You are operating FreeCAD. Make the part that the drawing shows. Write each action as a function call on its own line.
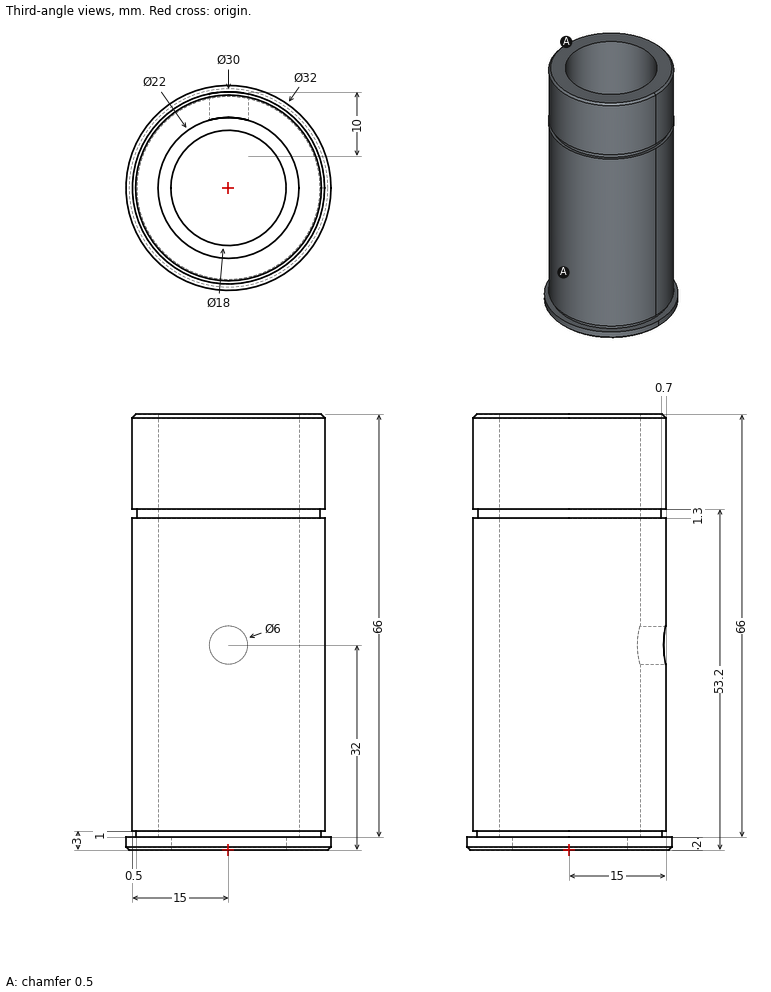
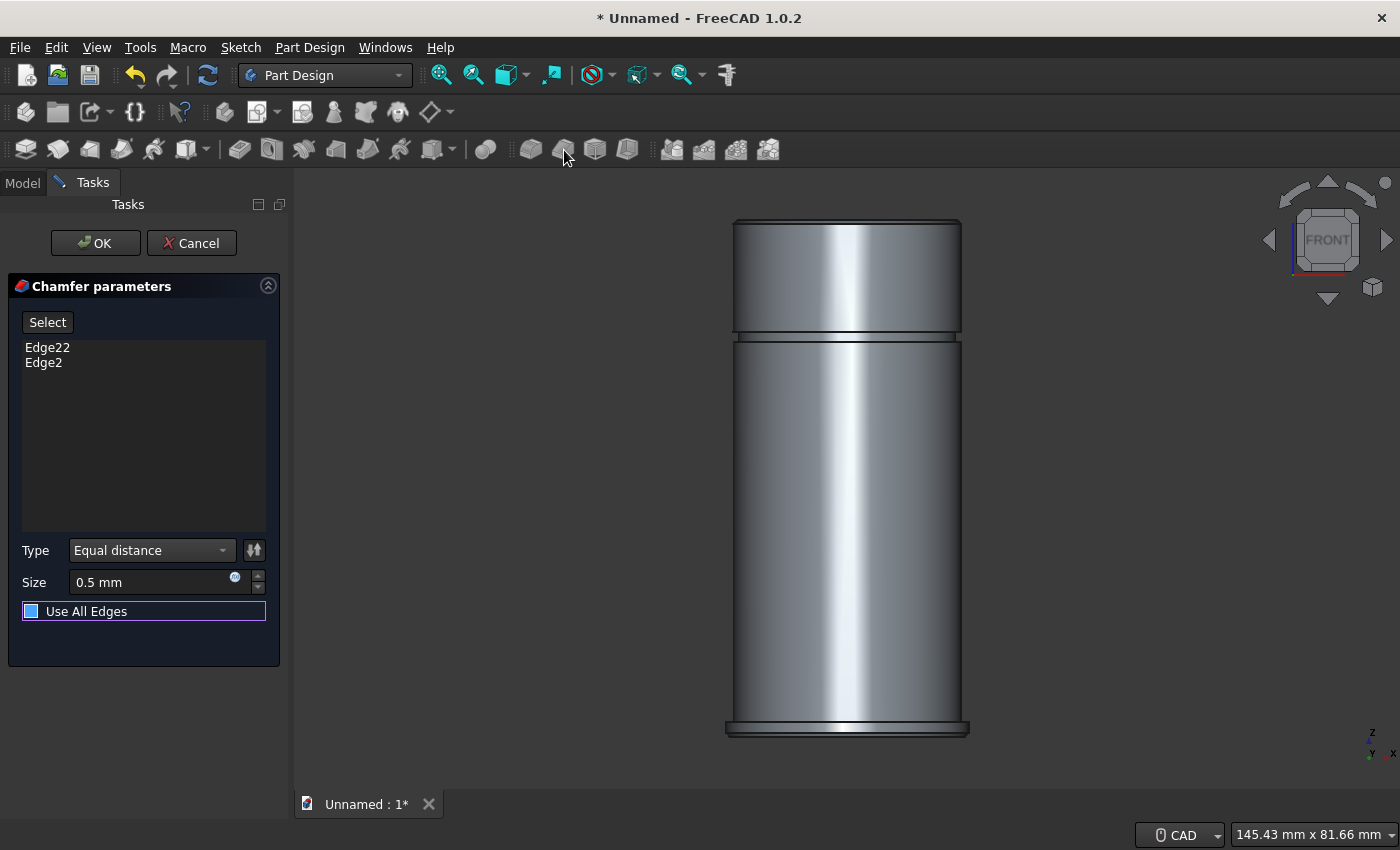
click(96, 243)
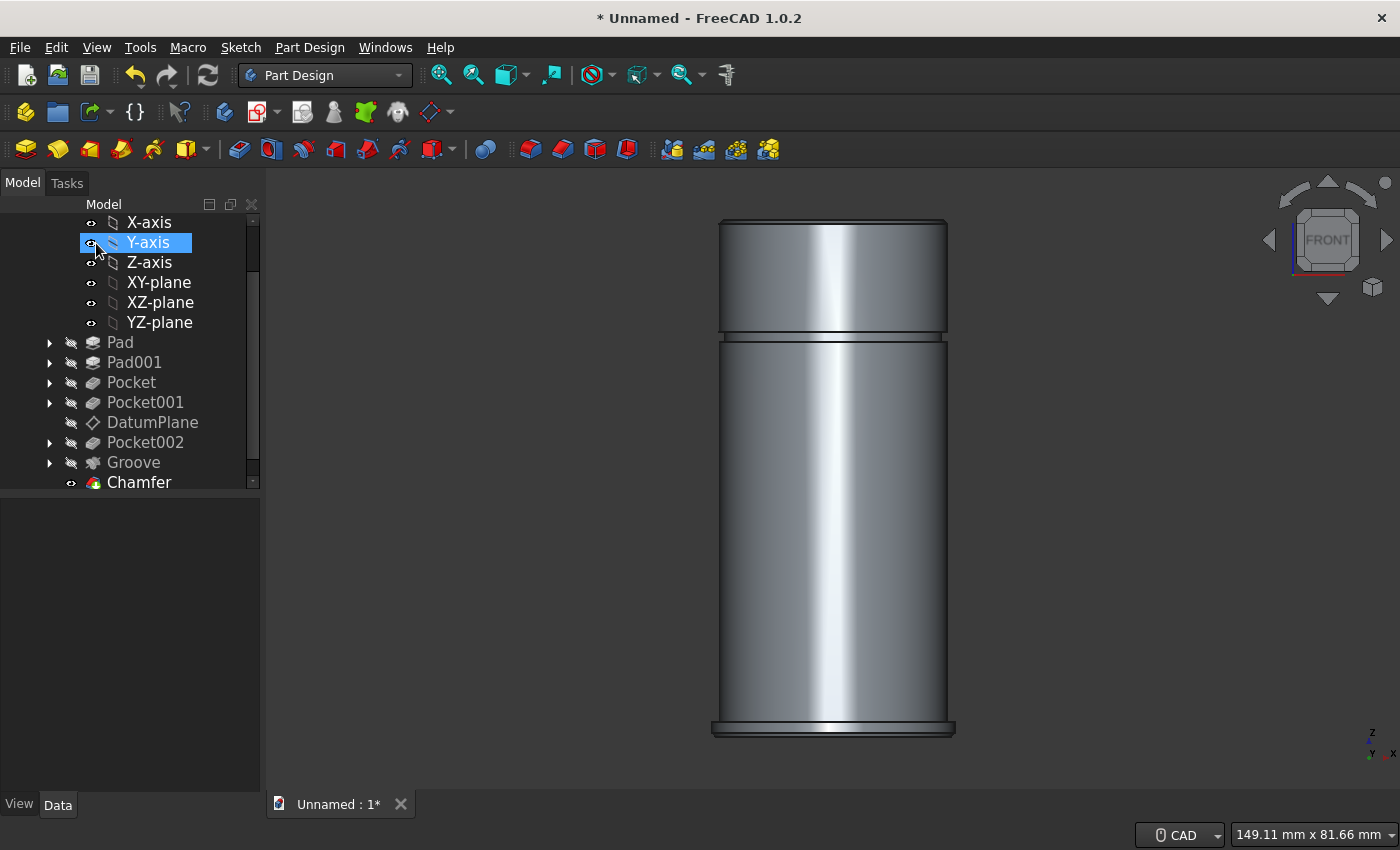
click(258, 112)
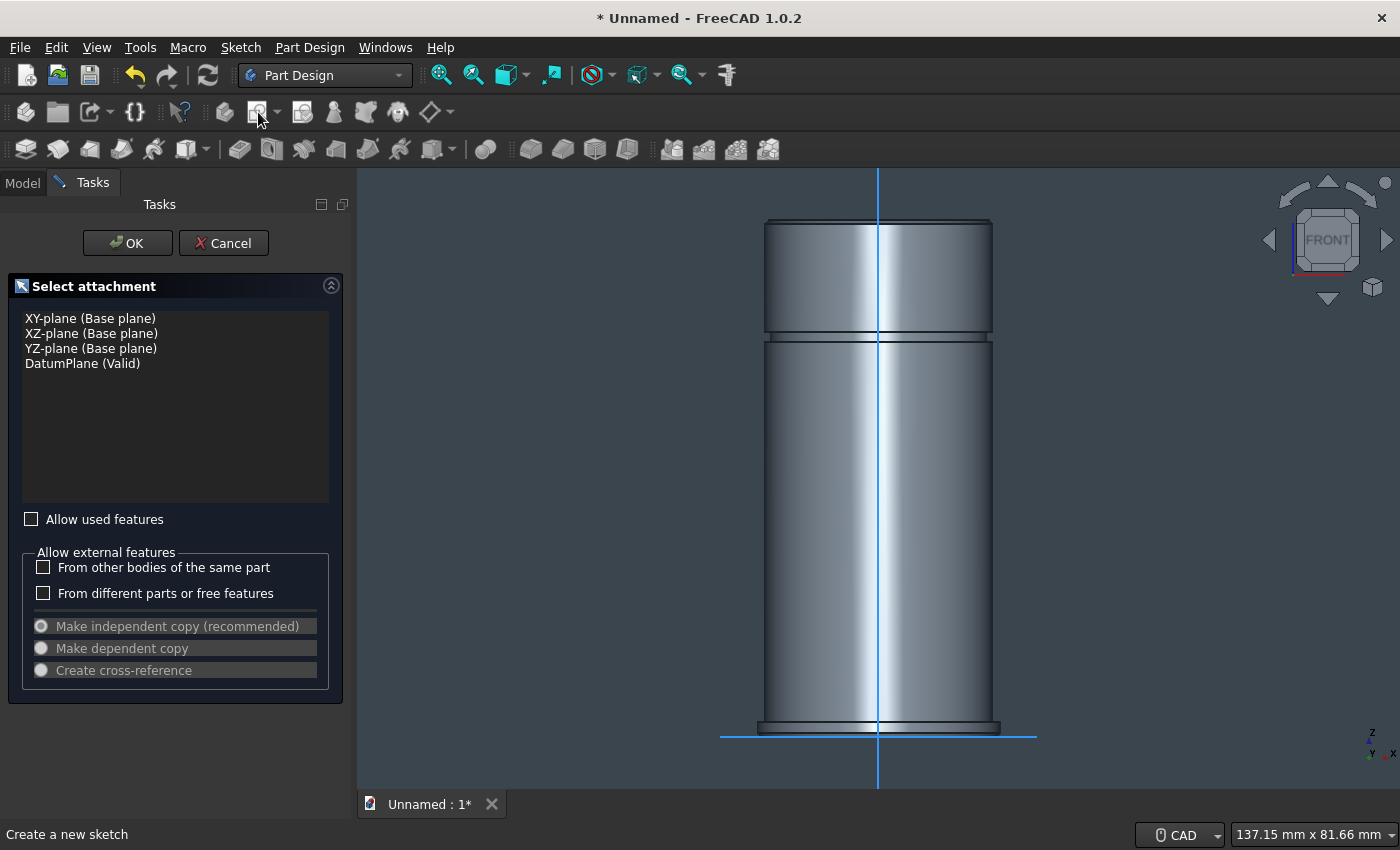
click(82, 334)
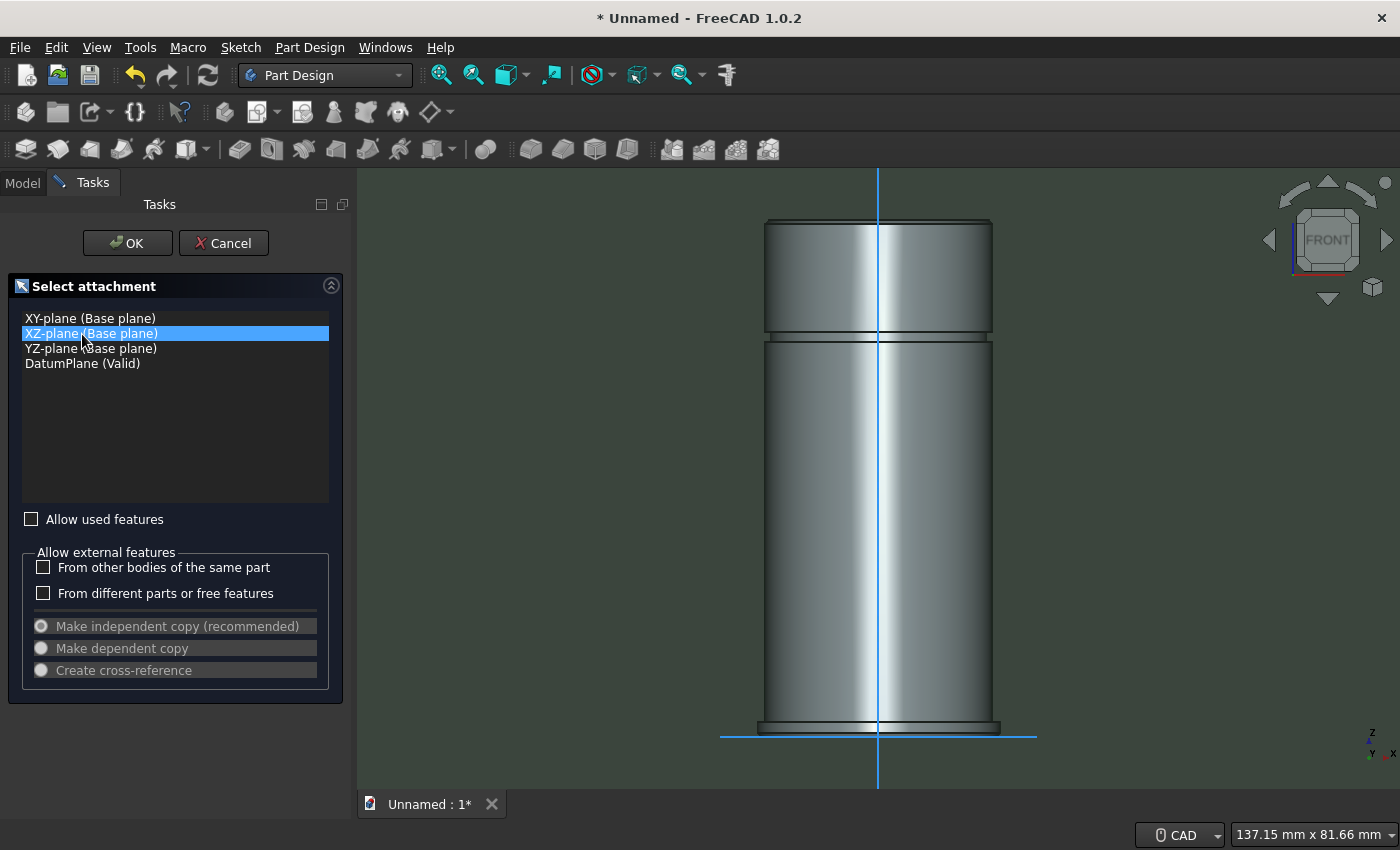
click(128, 243)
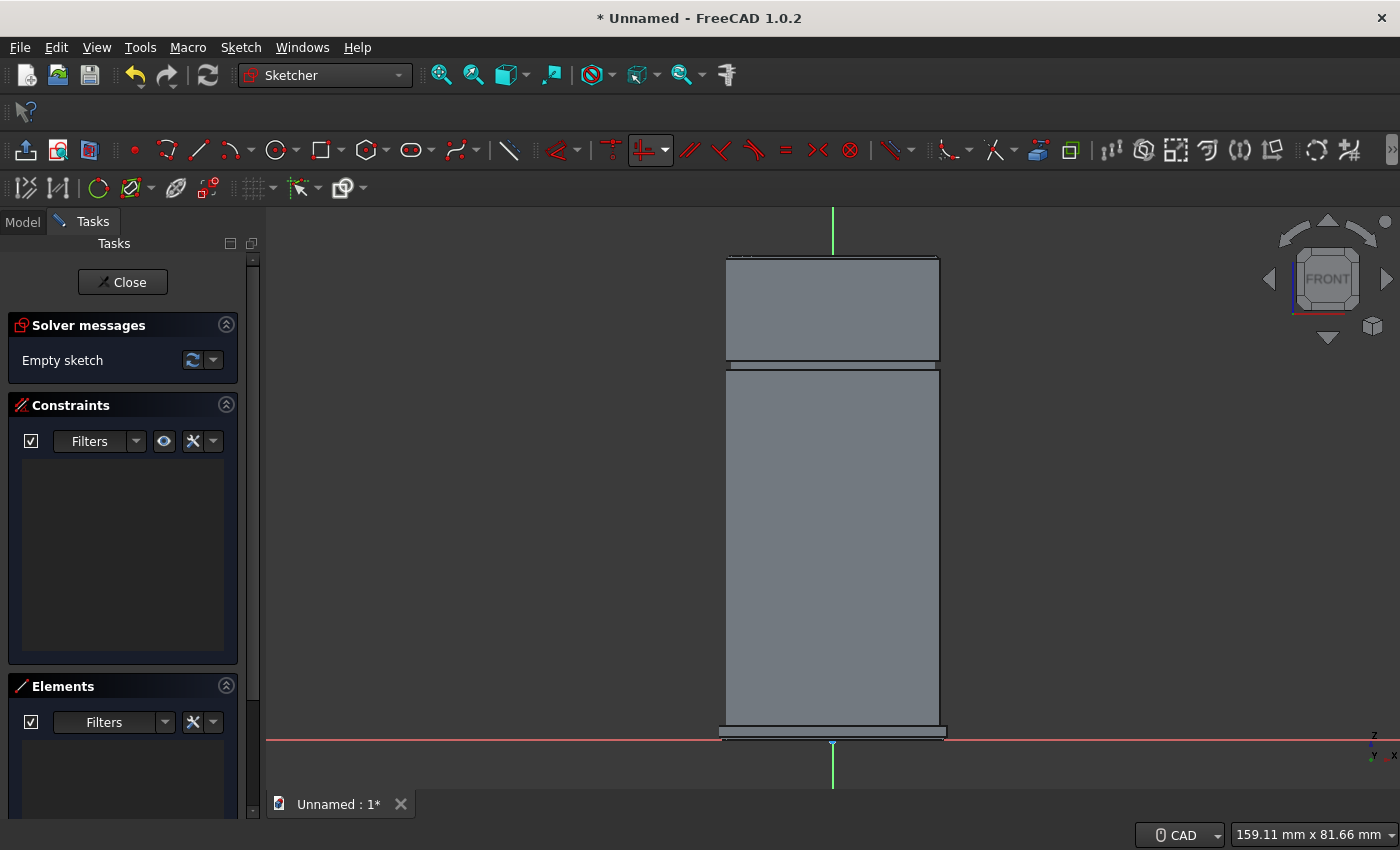
key(q)
key(s)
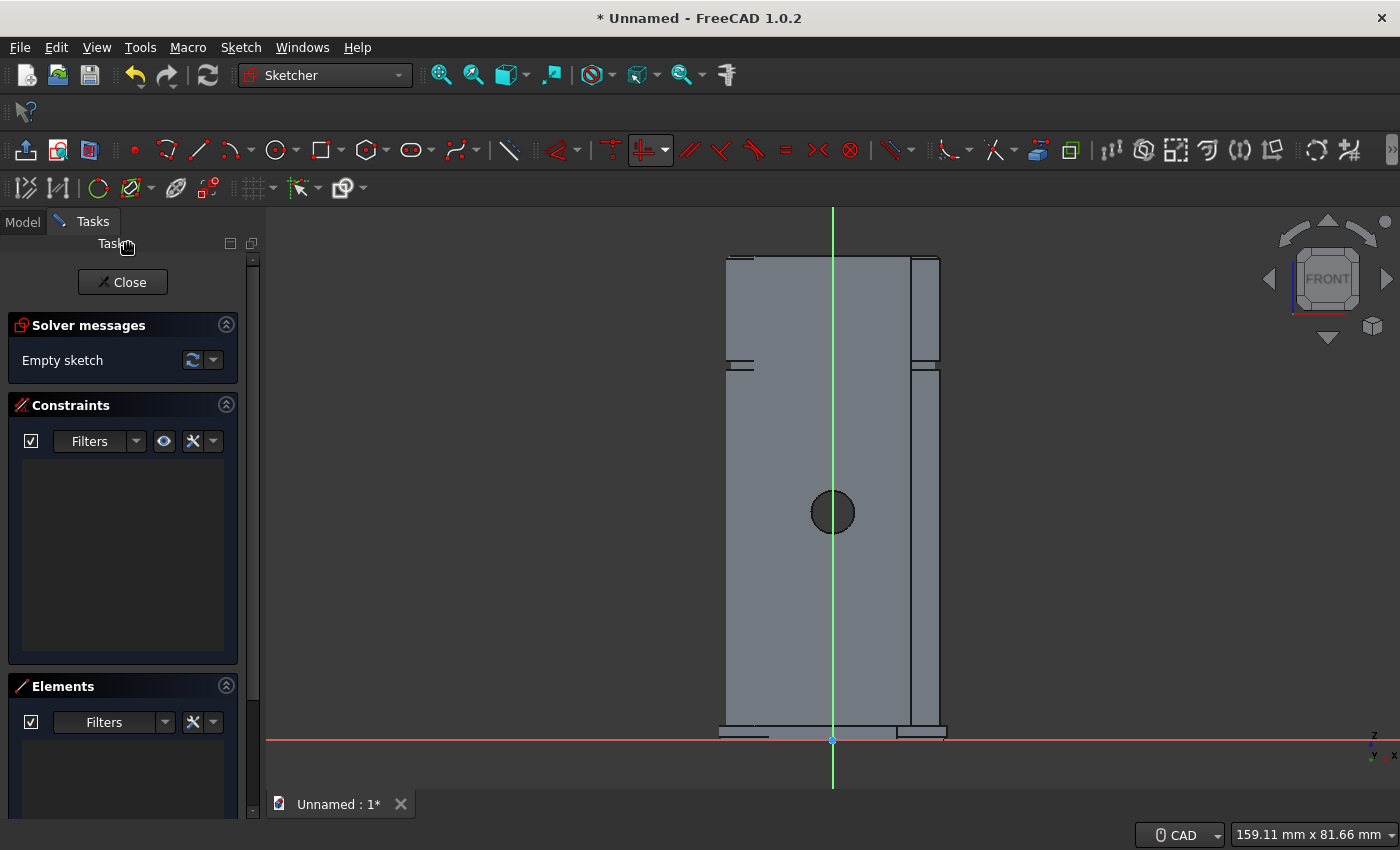
scroll(726, 734, up, 15)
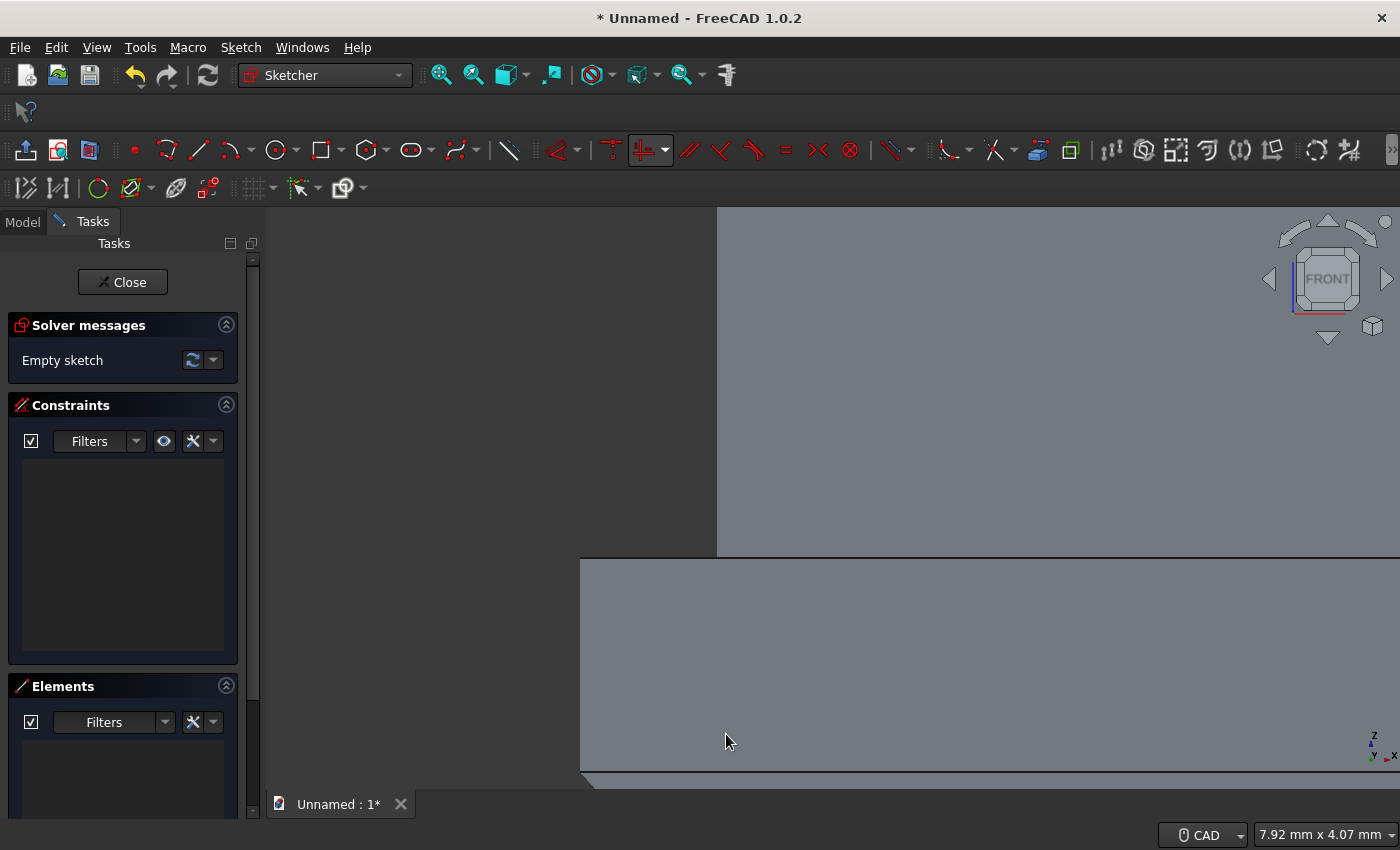
scroll(746, 479, up, 5)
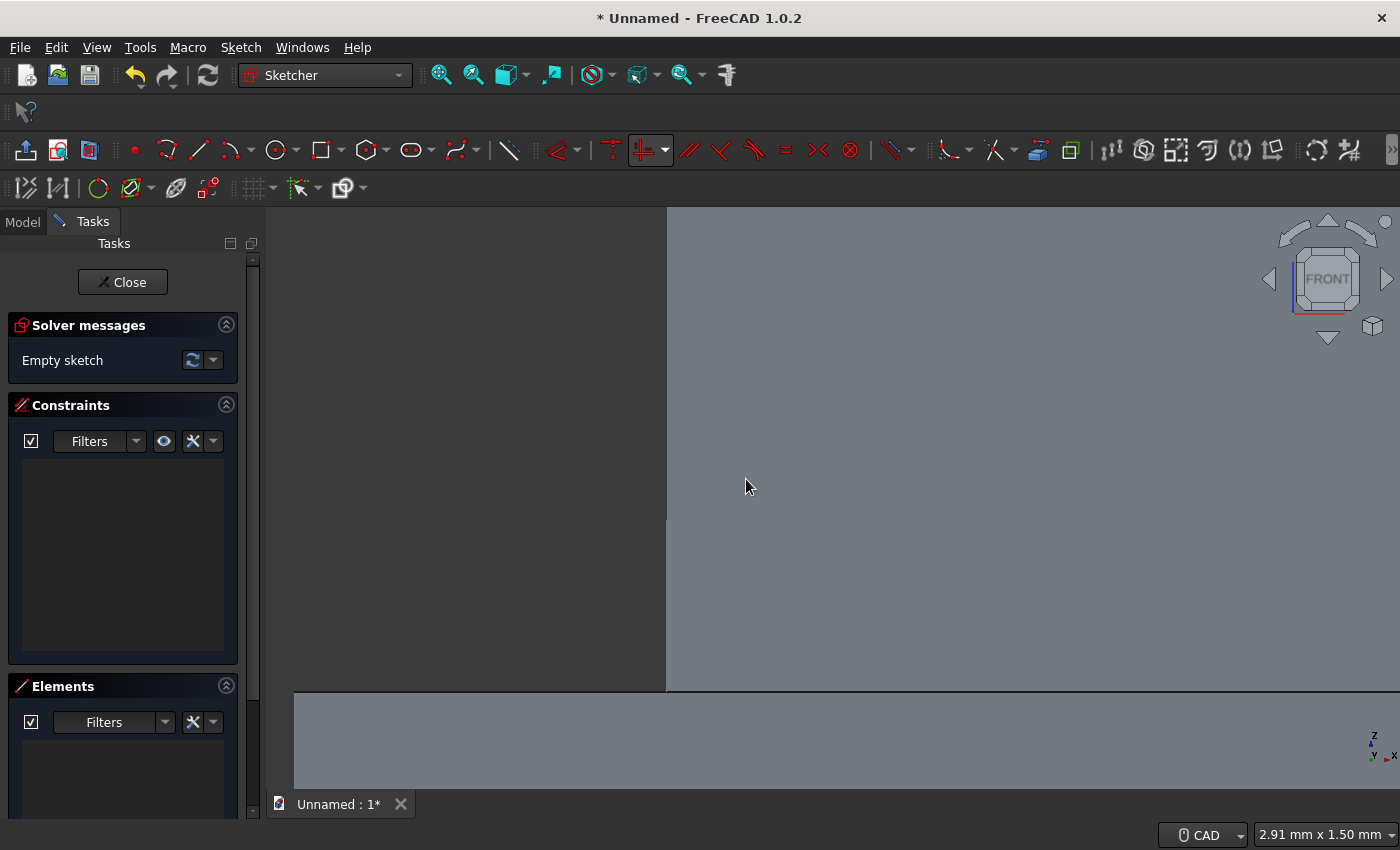
key(g)
key(r)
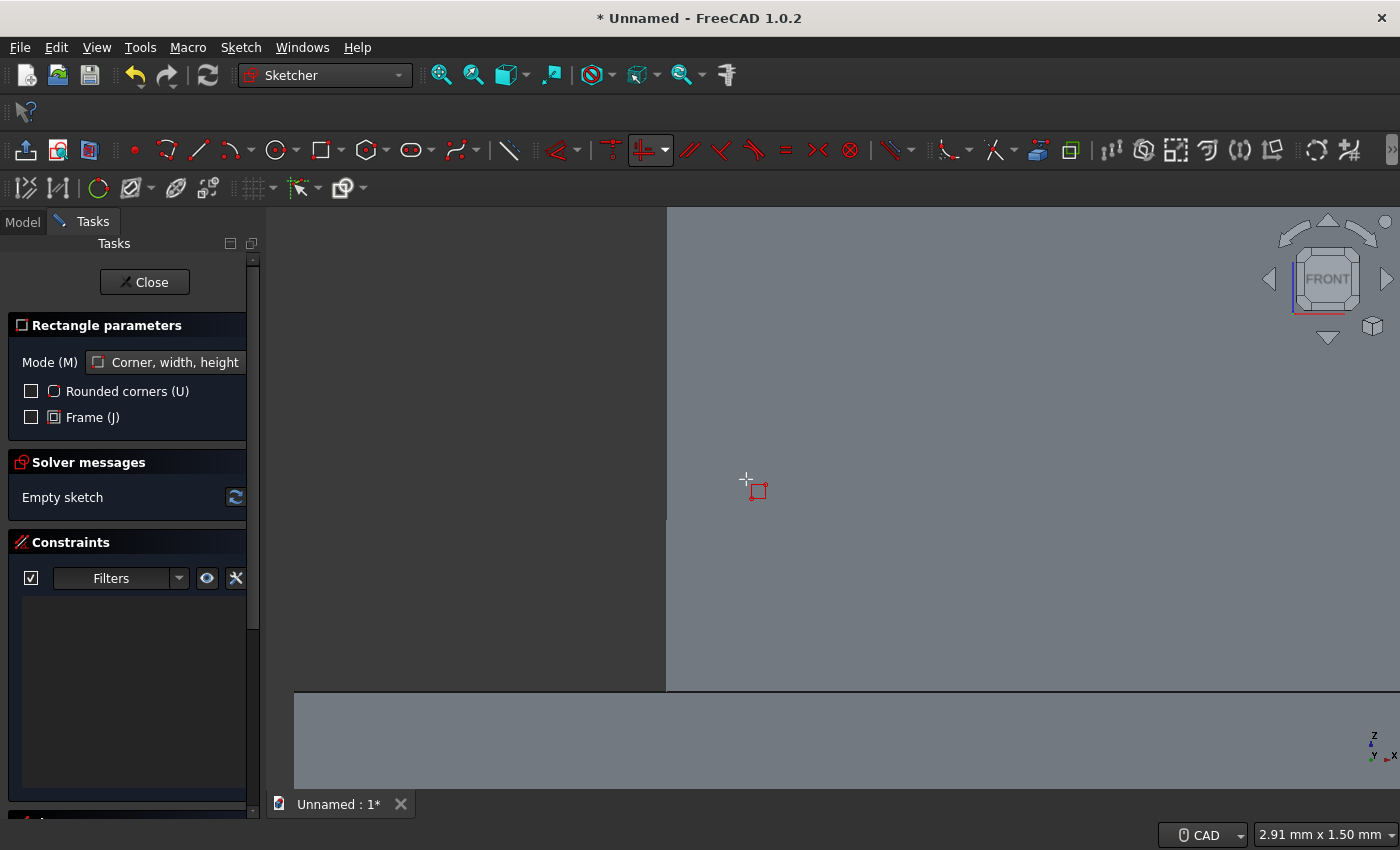
click(666, 302)
move(861, 692)